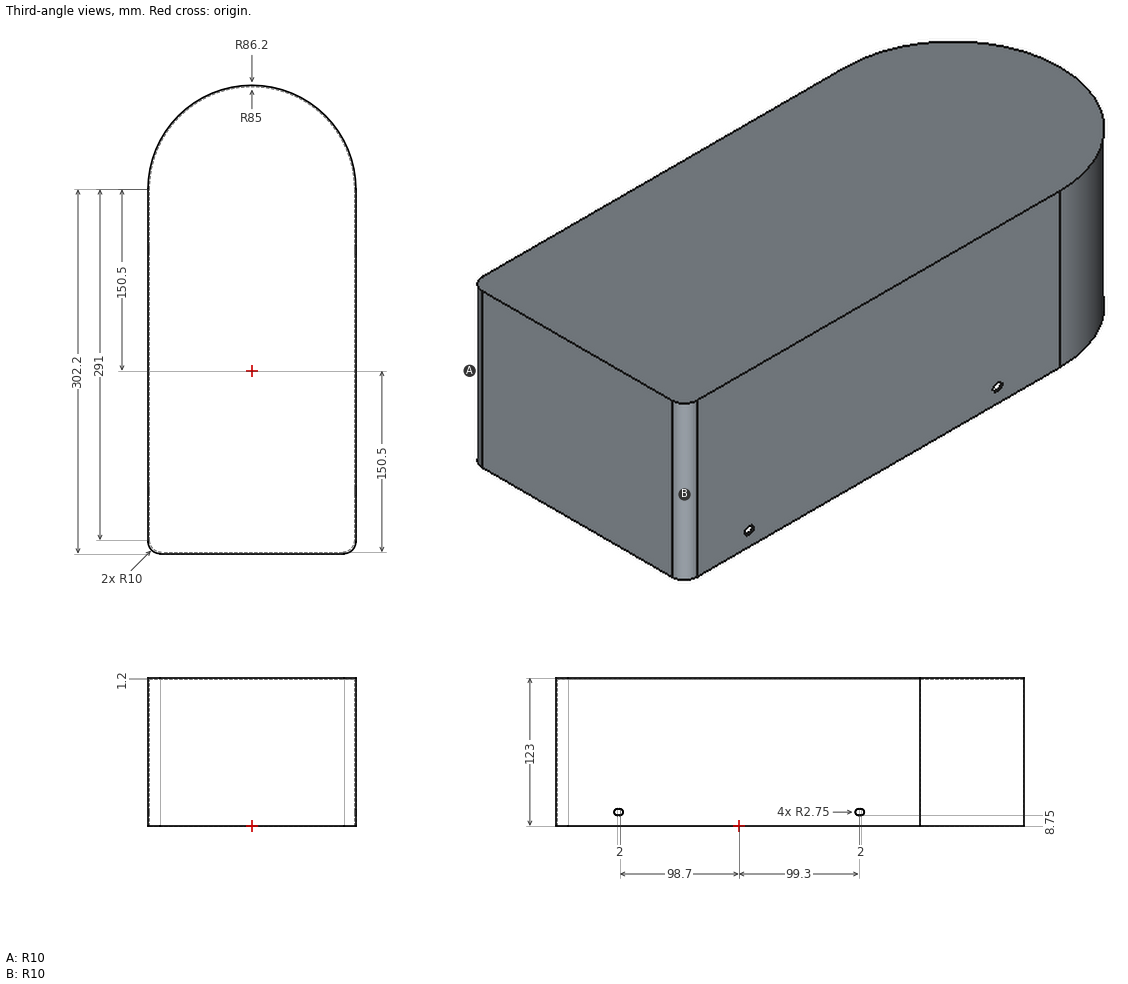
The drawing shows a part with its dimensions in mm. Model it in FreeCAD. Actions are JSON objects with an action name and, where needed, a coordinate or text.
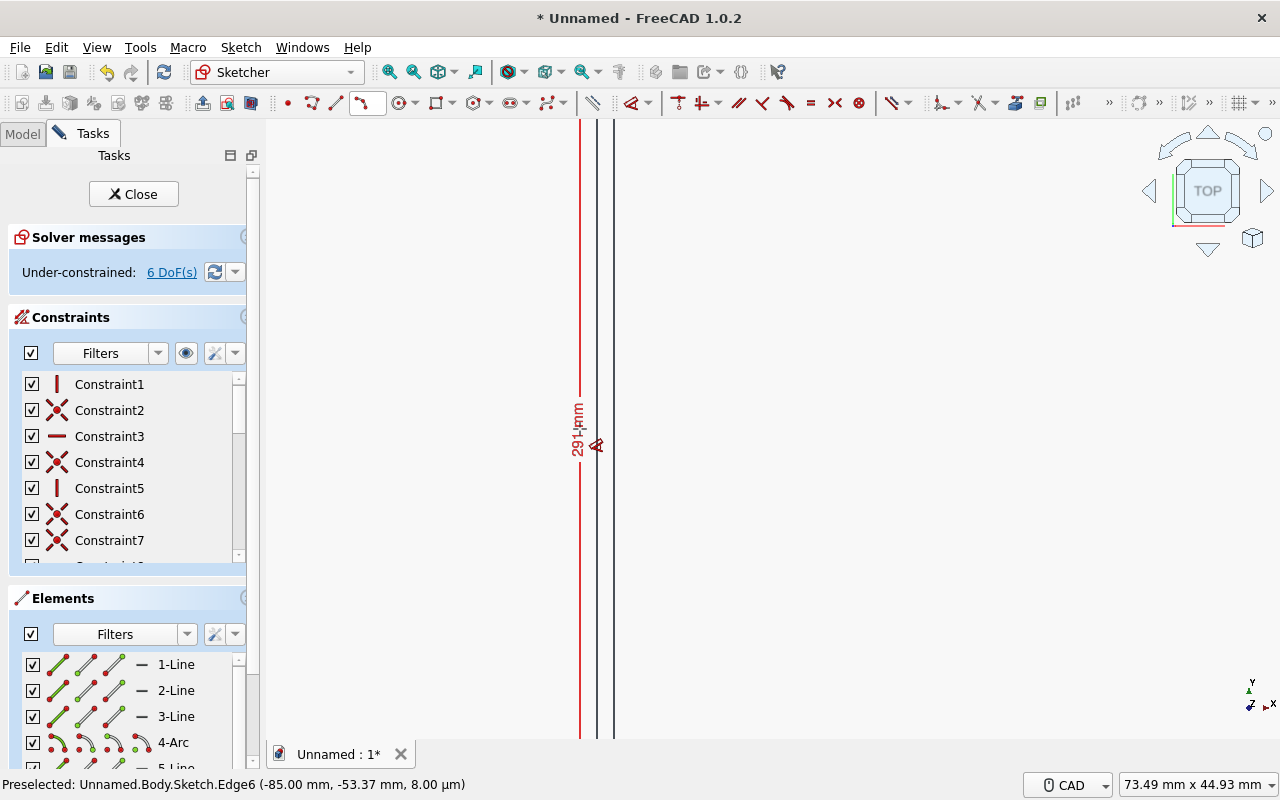
{"action": "scroll", "coordinate": [618, 527], "scroll_direction": "down", "scroll_amount": 13}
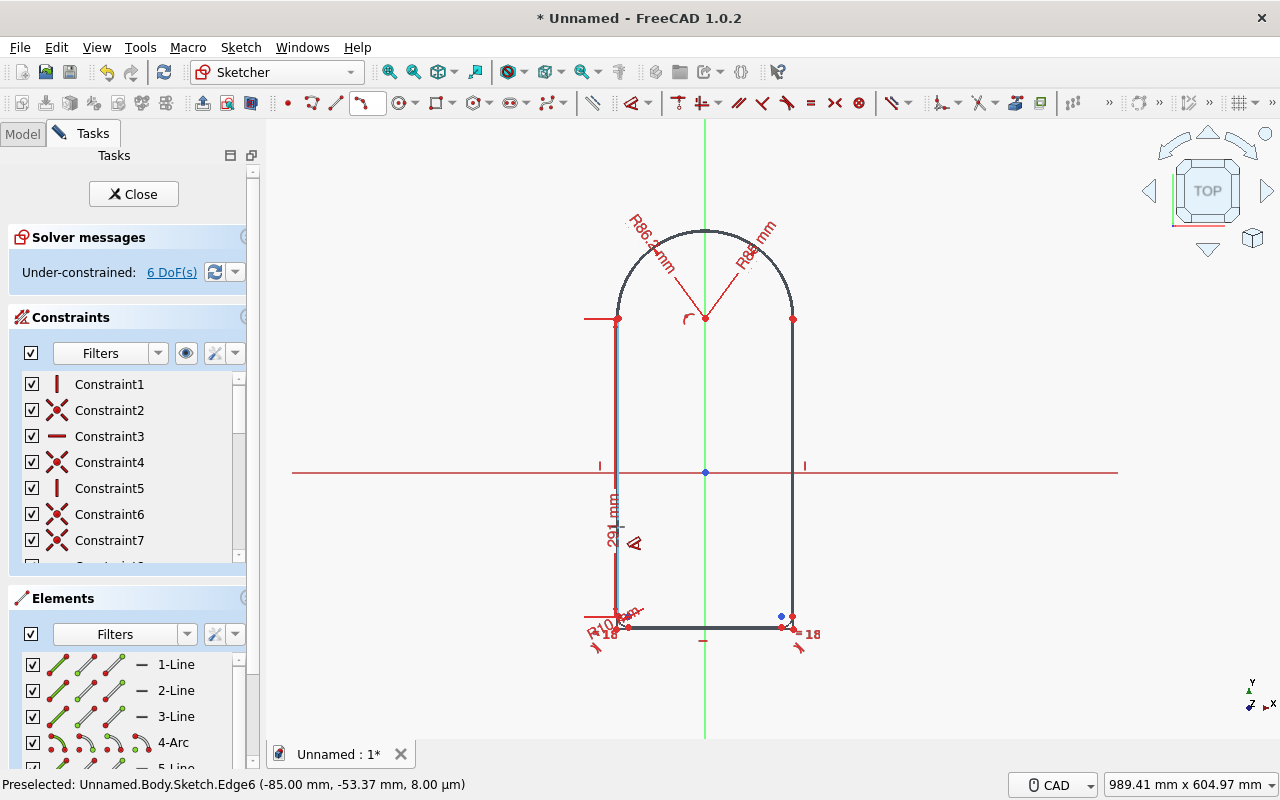
{"action": "scroll", "coordinate": [792, 408], "scroll_direction": "up", "scroll_amount": 13}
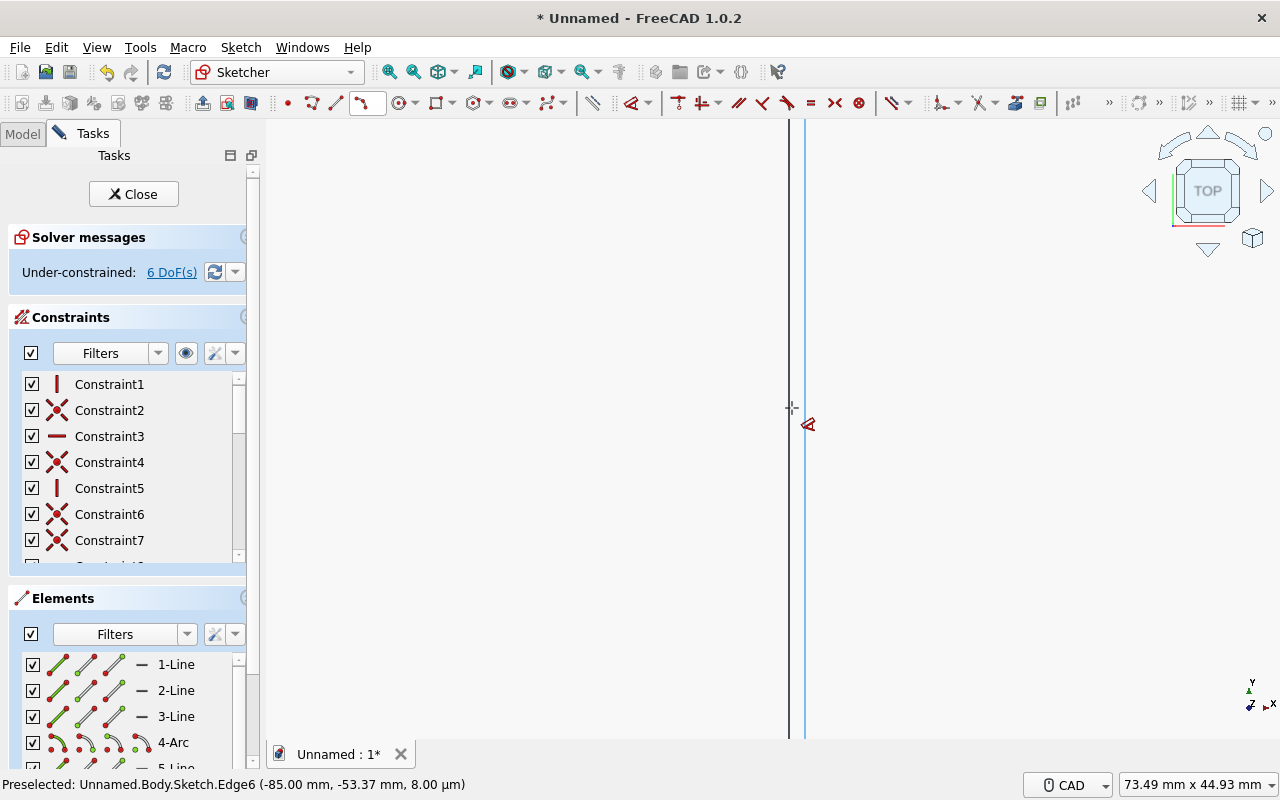
{"action": "left_click", "coordinate": [789, 404]}
{"action": "left_click", "coordinate": [823, 429]}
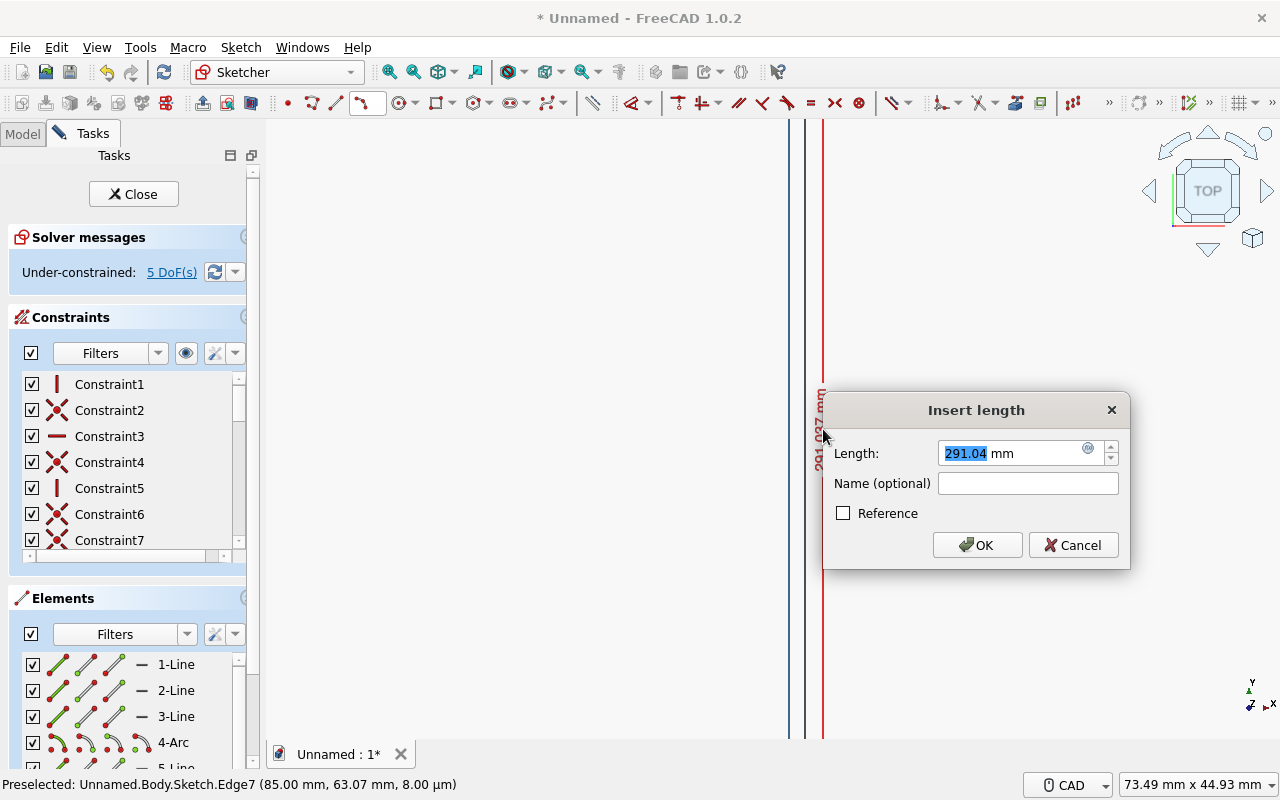
{"action": "type", "text": "291"}
{"action": "key", "text": "Return"}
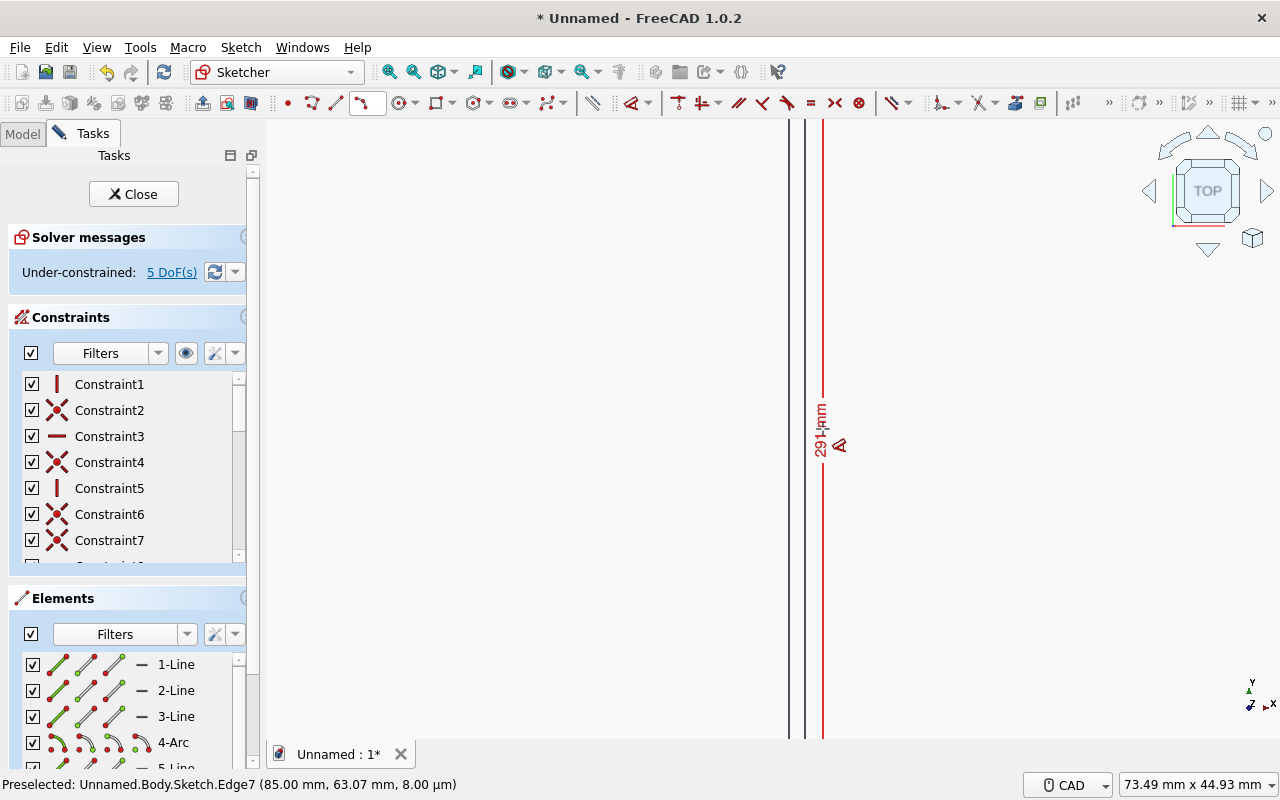
{"action": "scroll", "coordinate": [792, 408], "scroll_direction": "down", "scroll_amount": 13}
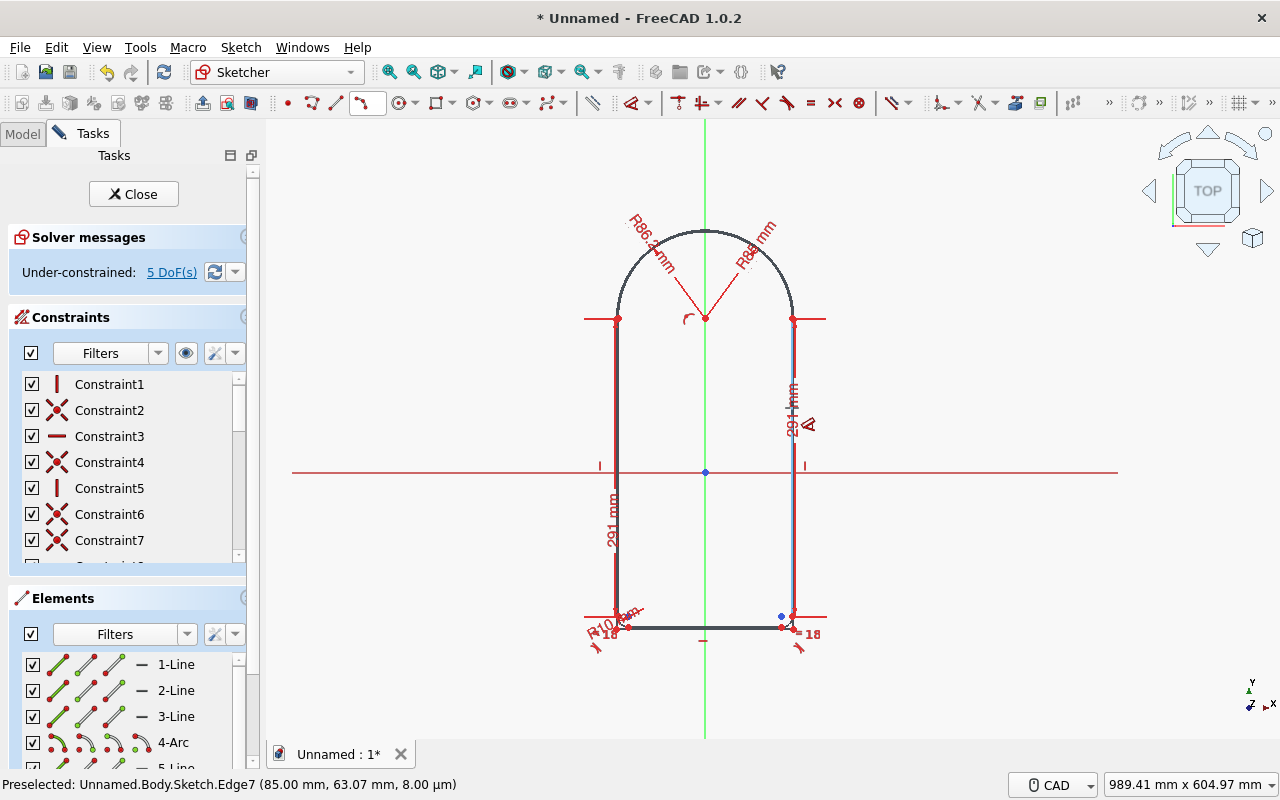
{"action": "scroll", "coordinate": [617, 412], "scroll_direction": "up", "scroll_amount": 13}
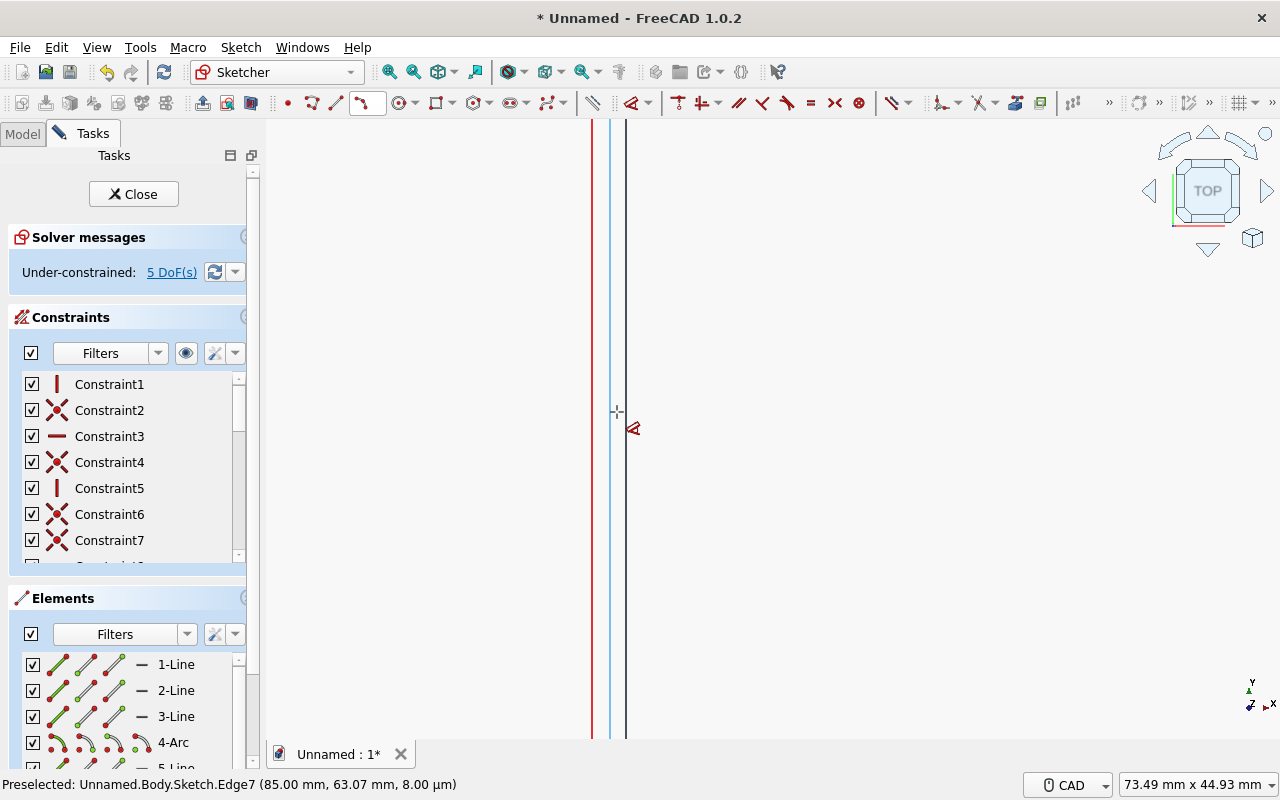
{"action": "left_click", "coordinate": [610, 412]}
{"action": "left_click", "coordinate": [576, 429]}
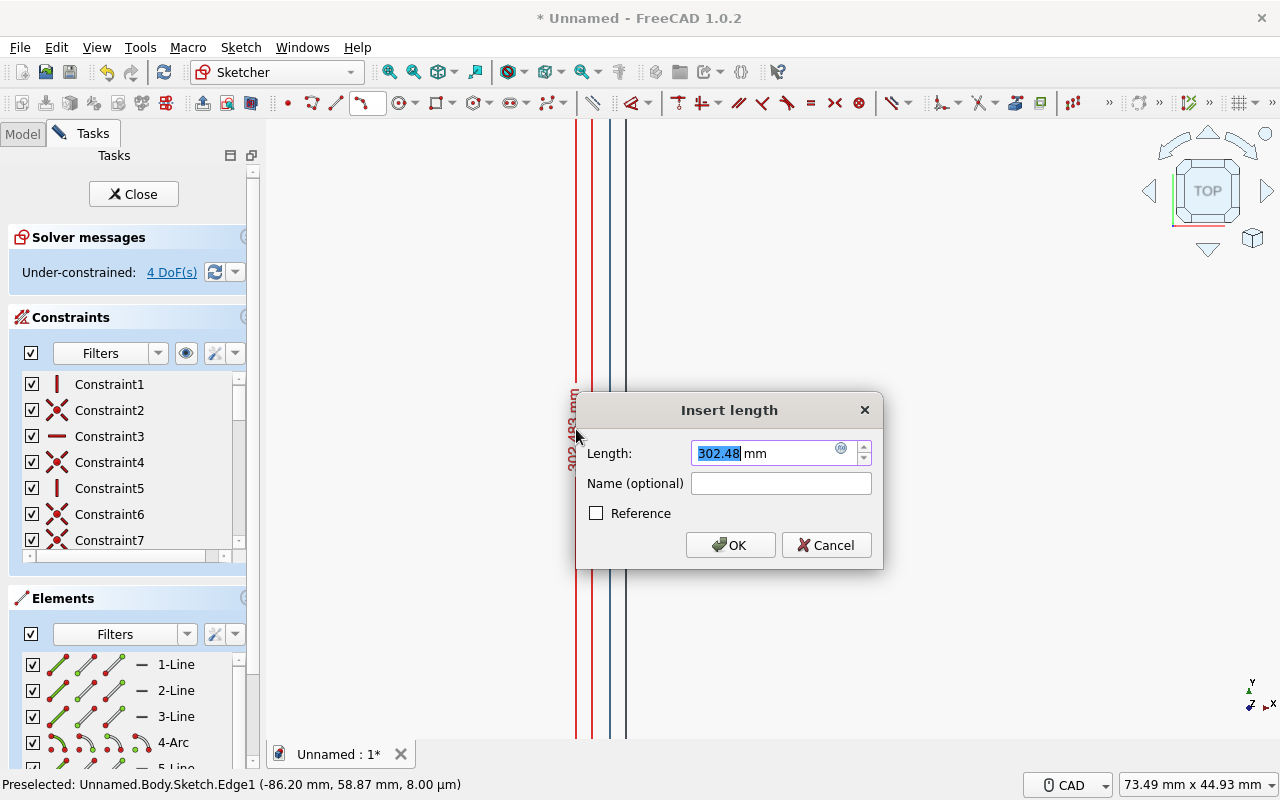
{"action": "type", "text": "302.2"}
{"action": "key", "text": "Return"}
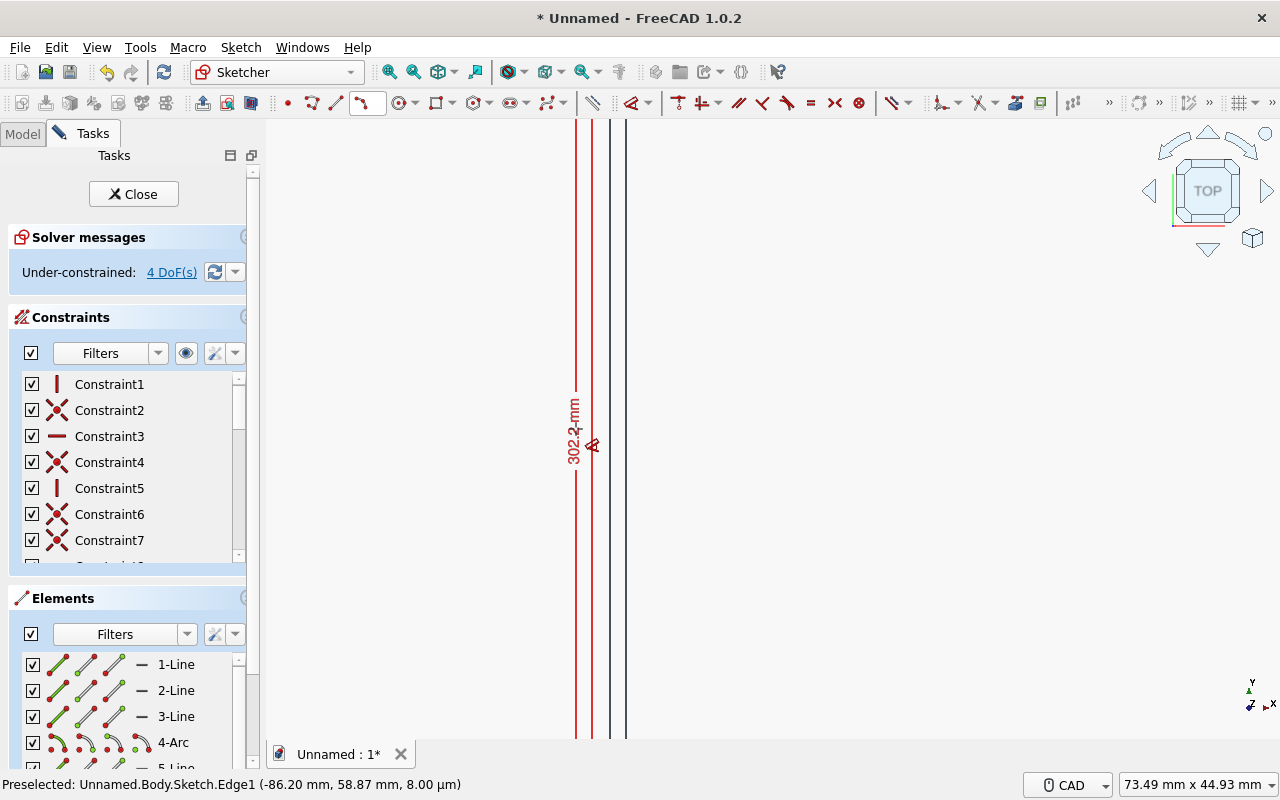
{"action": "scroll", "coordinate": [617, 412], "scroll_direction": "down", "scroll_amount": 13}